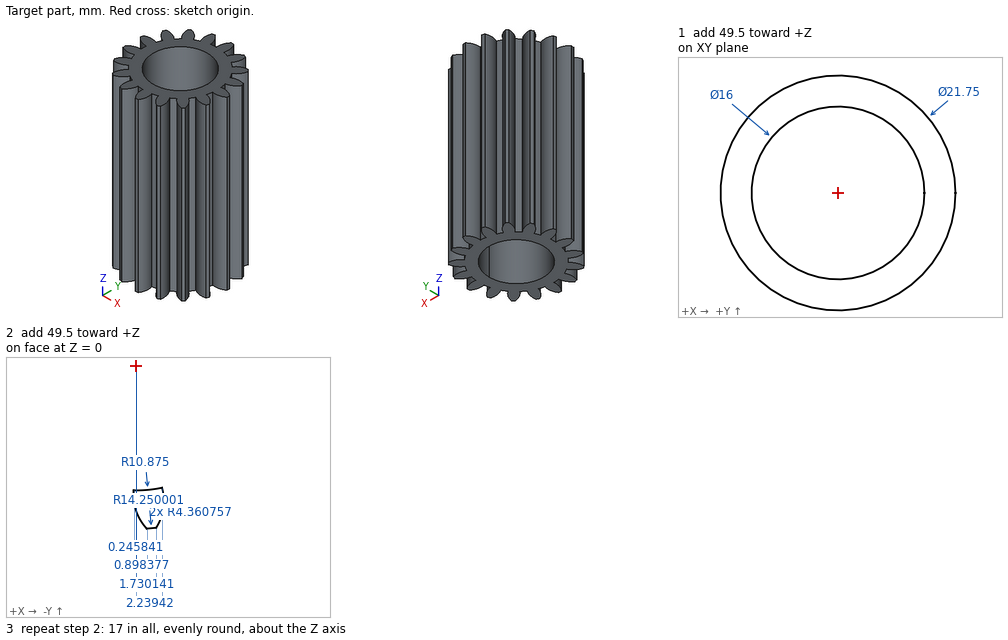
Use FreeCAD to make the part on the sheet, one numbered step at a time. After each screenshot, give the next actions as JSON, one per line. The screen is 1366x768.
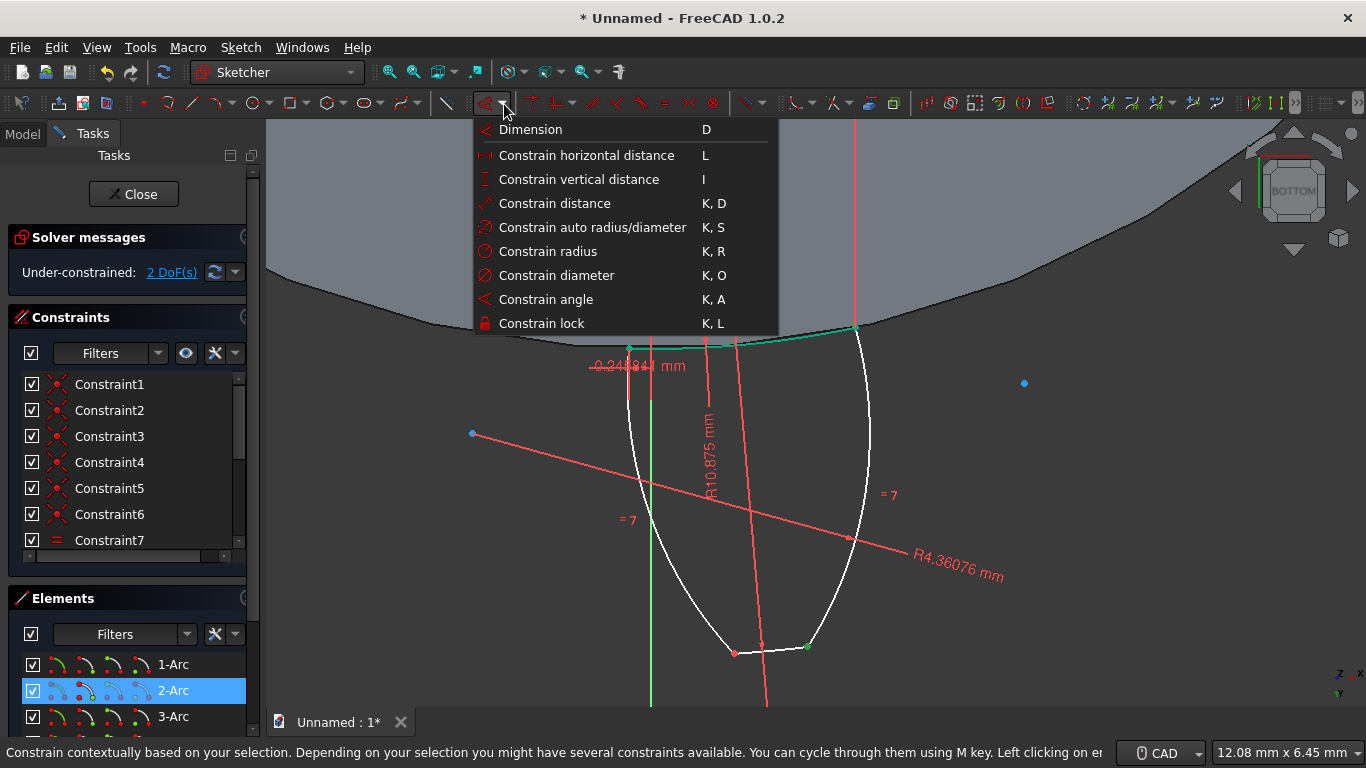
{"action": "left_click", "coordinate": [626, 155]}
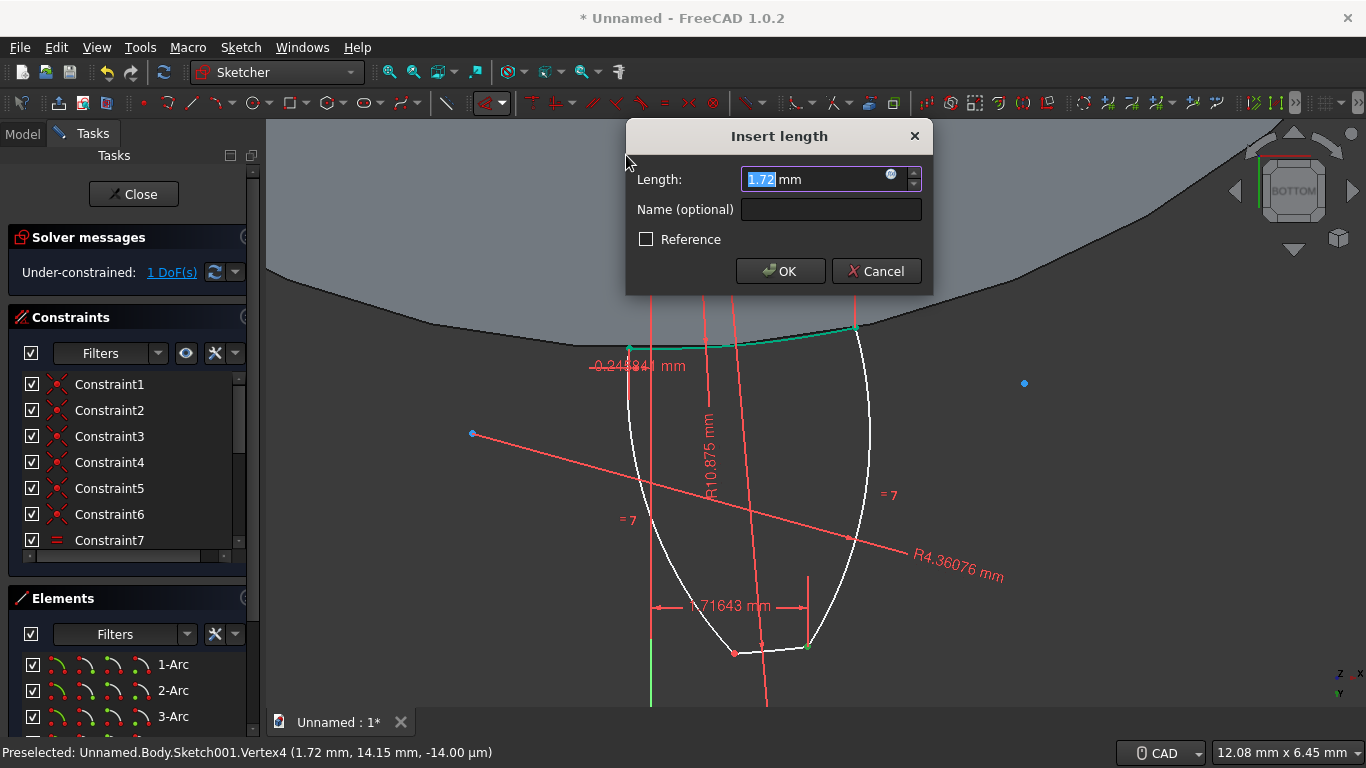
{"action": "type", "text": "1.730141"}
{"action": "key", "text": "Return"}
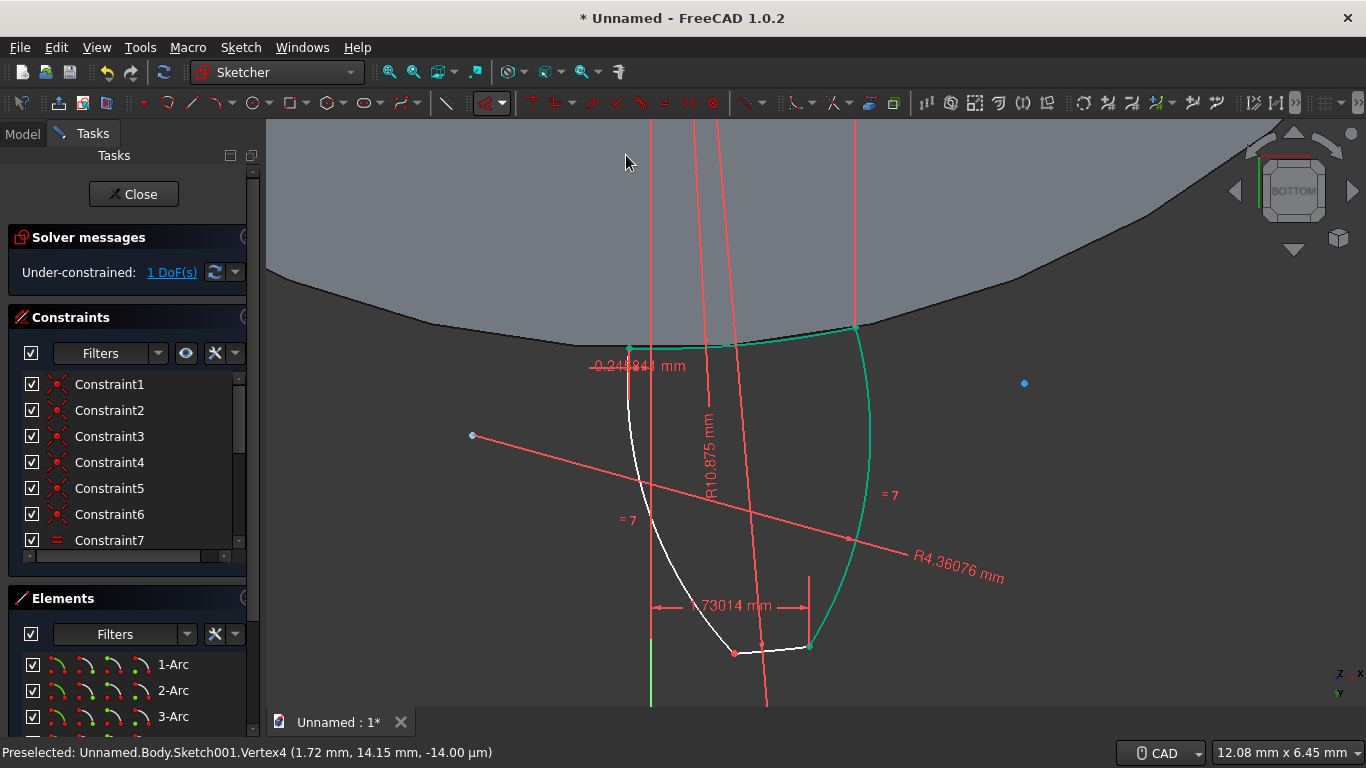
{"action": "left_click", "coordinate": [734, 654]}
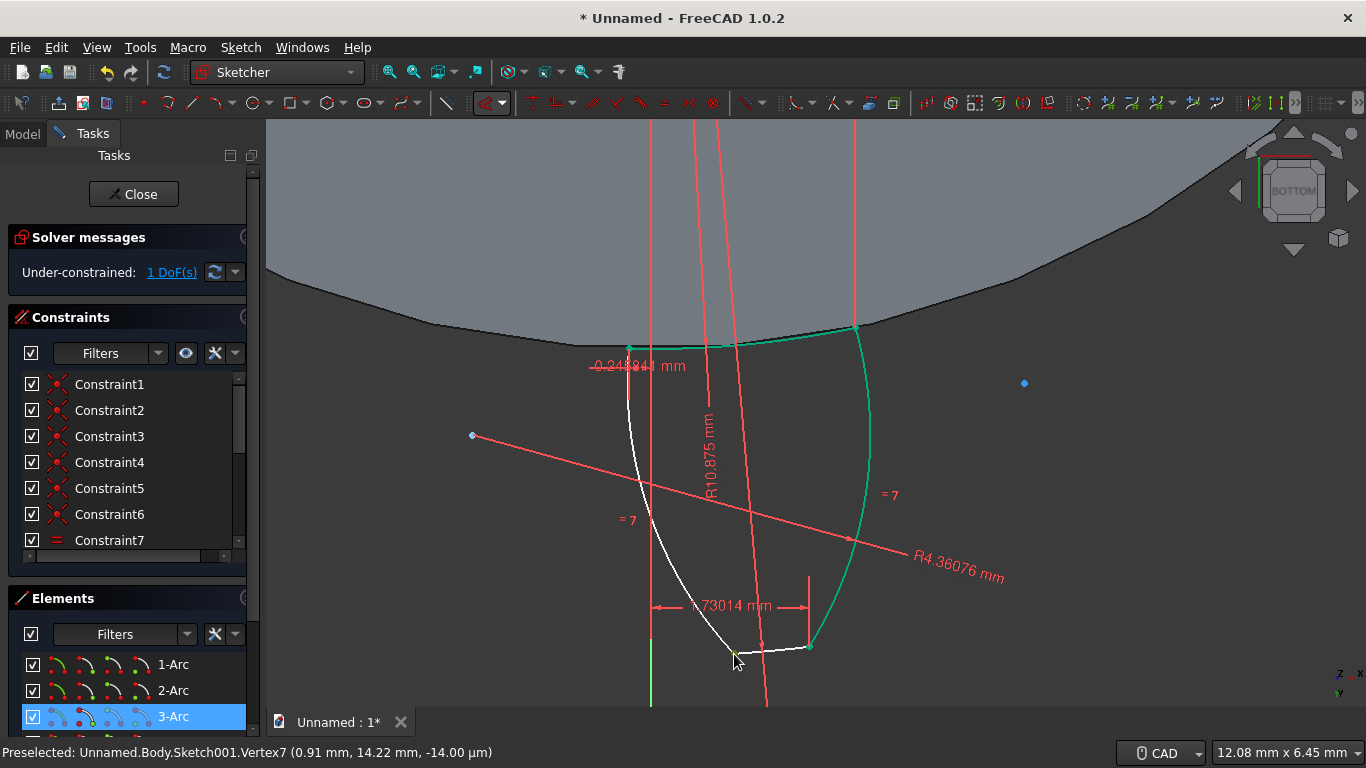
{"action": "left_click", "coordinate": [504, 104]}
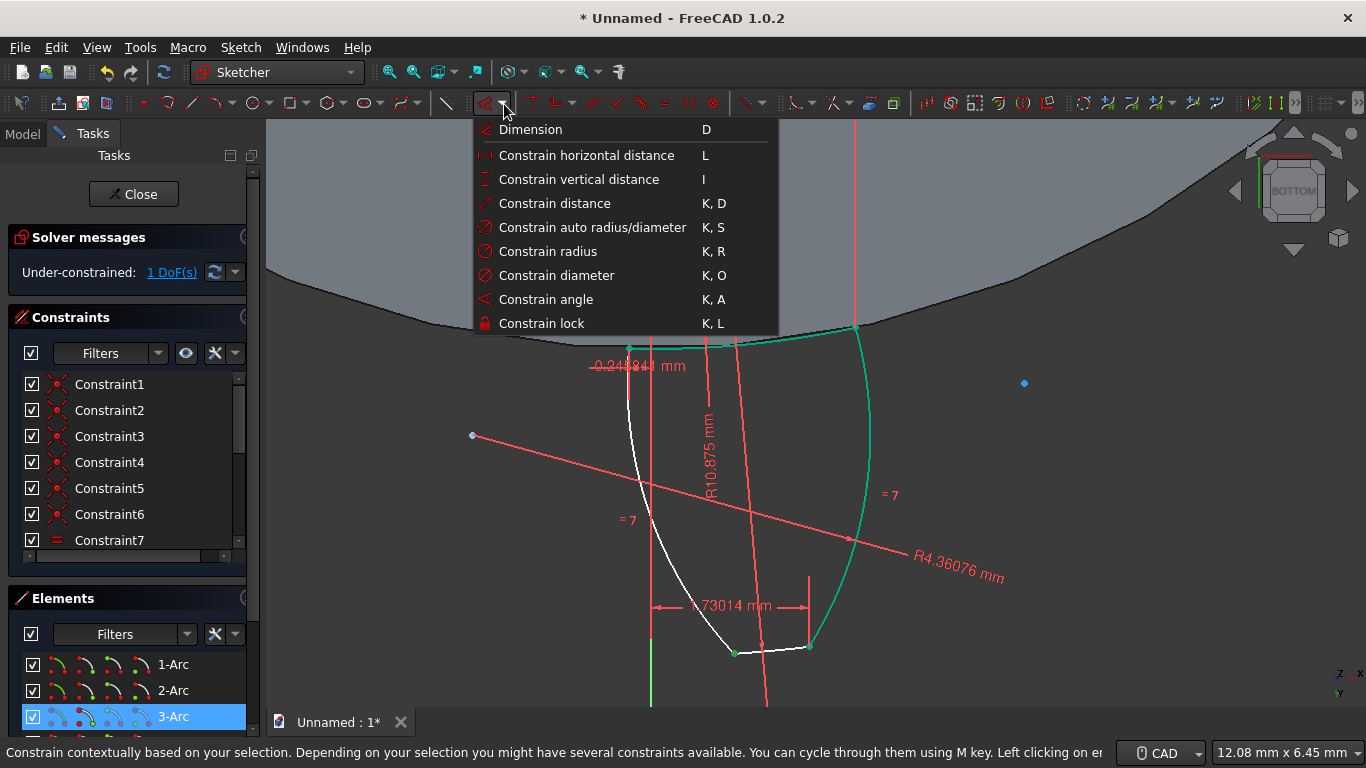
{"action": "left_click", "coordinate": [626, 155]}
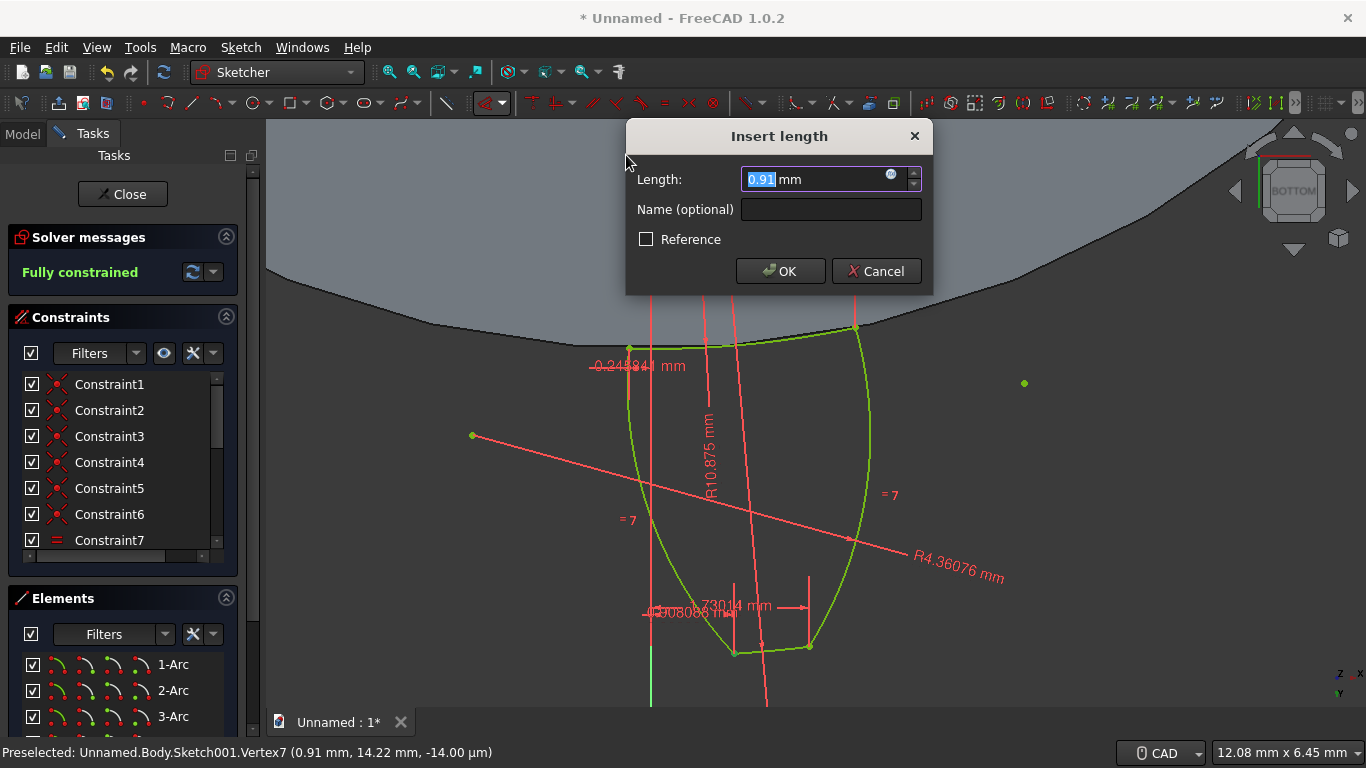
{"action": "type", "text": "0.898377"}
{"action": "key", "text": "Return"}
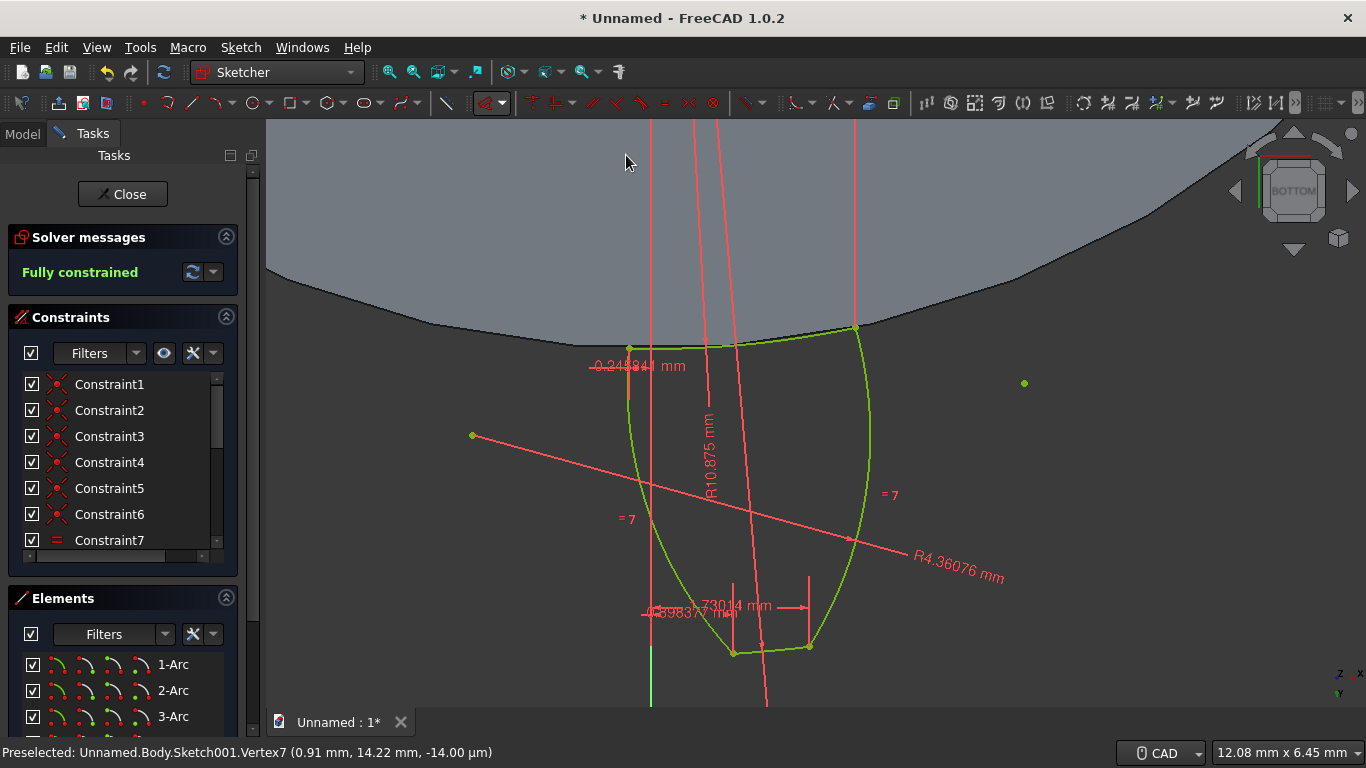
{"action": "left_click", "coordinate": [123, 194]}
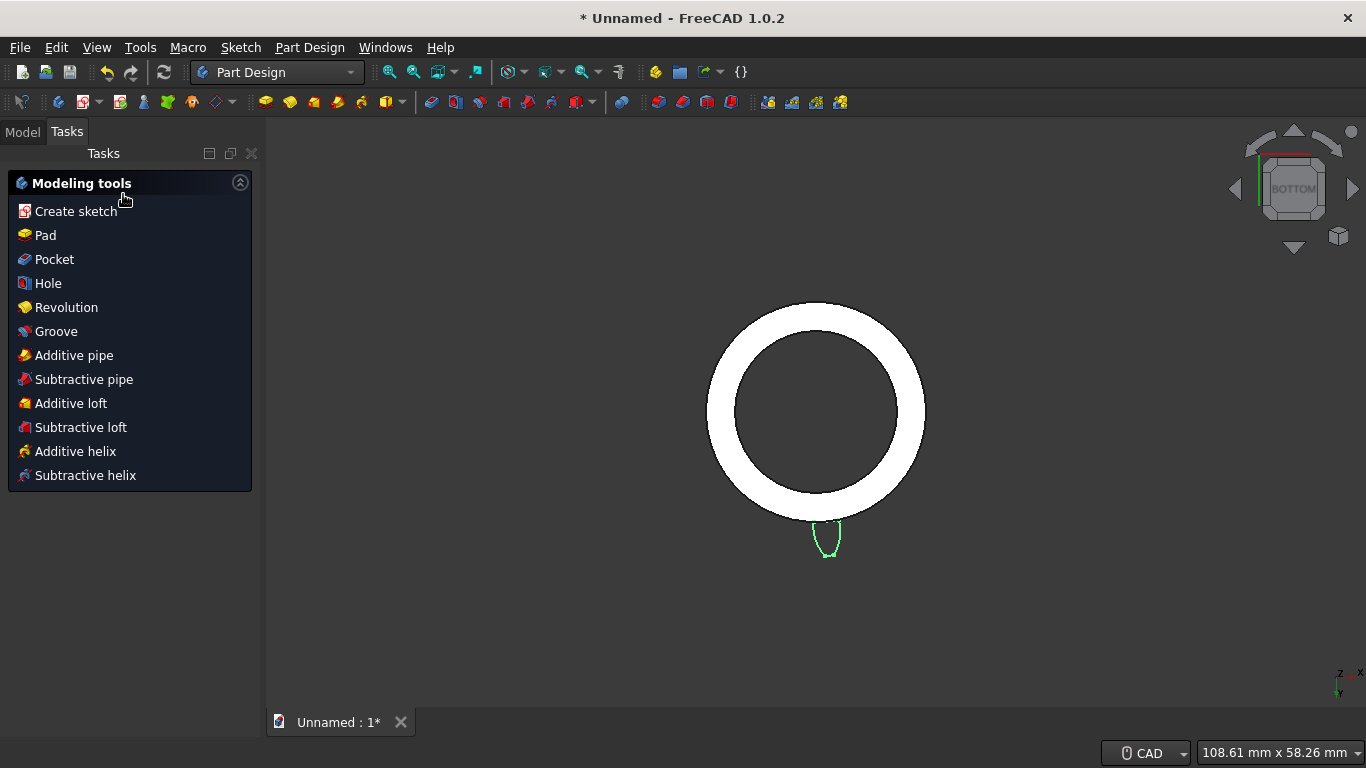
{"action": "left_click", "coordinate": [266, 102]}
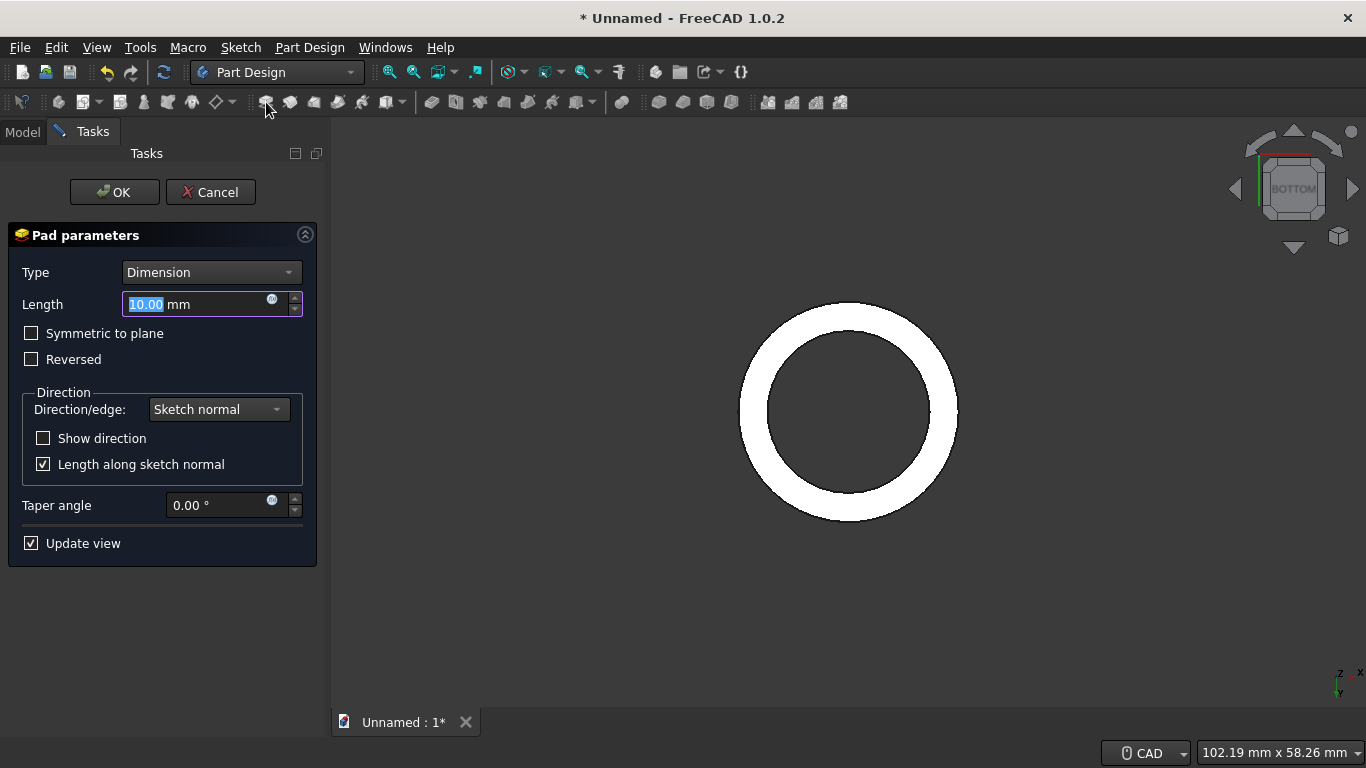
{"action": "type", "text": "49.5"}
{"action": "key", "text": "Tab"}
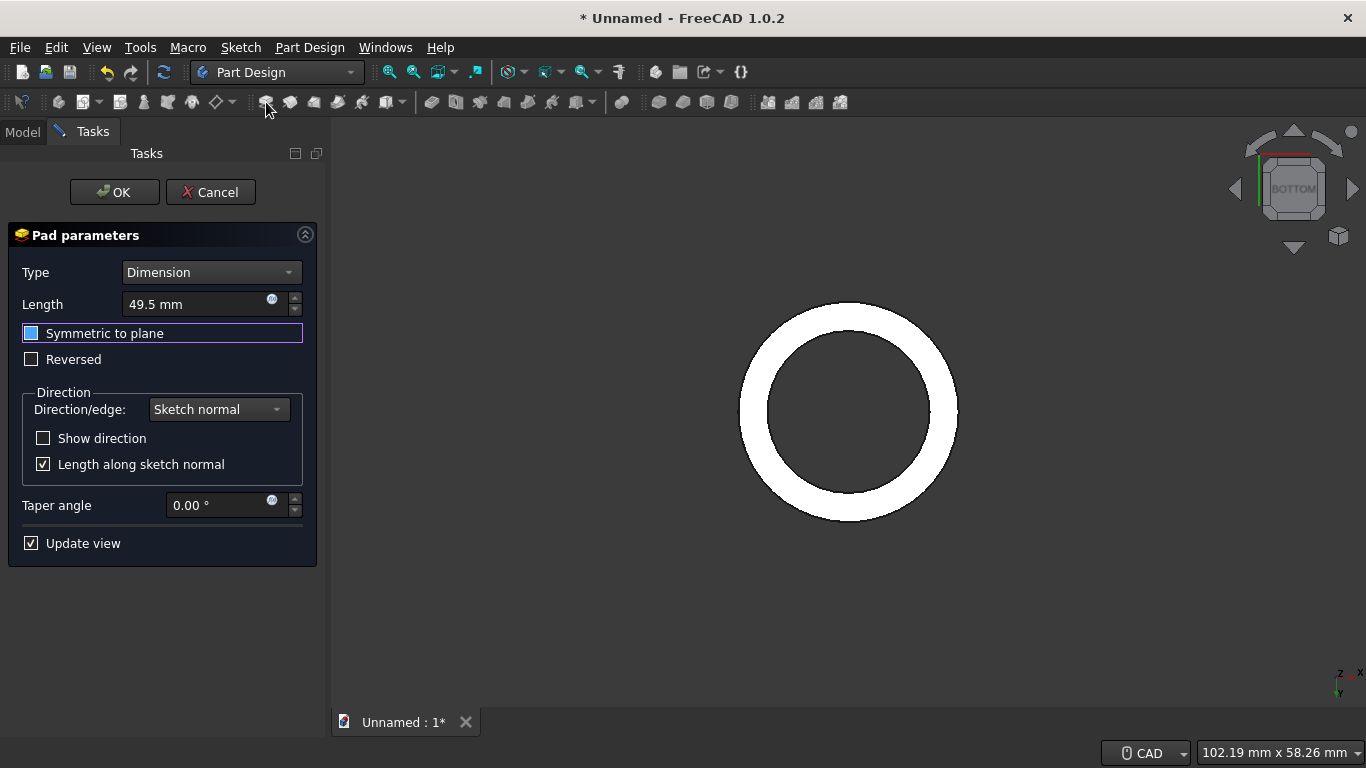
{"action": "left_click", "coordinate": [30, 359]}